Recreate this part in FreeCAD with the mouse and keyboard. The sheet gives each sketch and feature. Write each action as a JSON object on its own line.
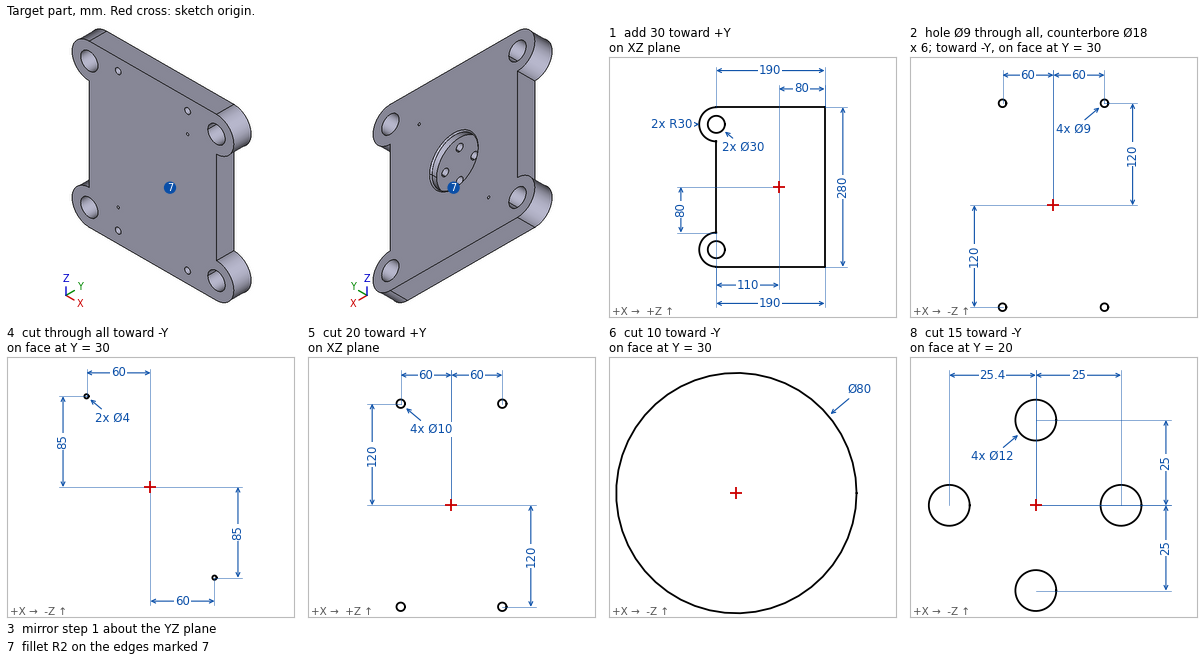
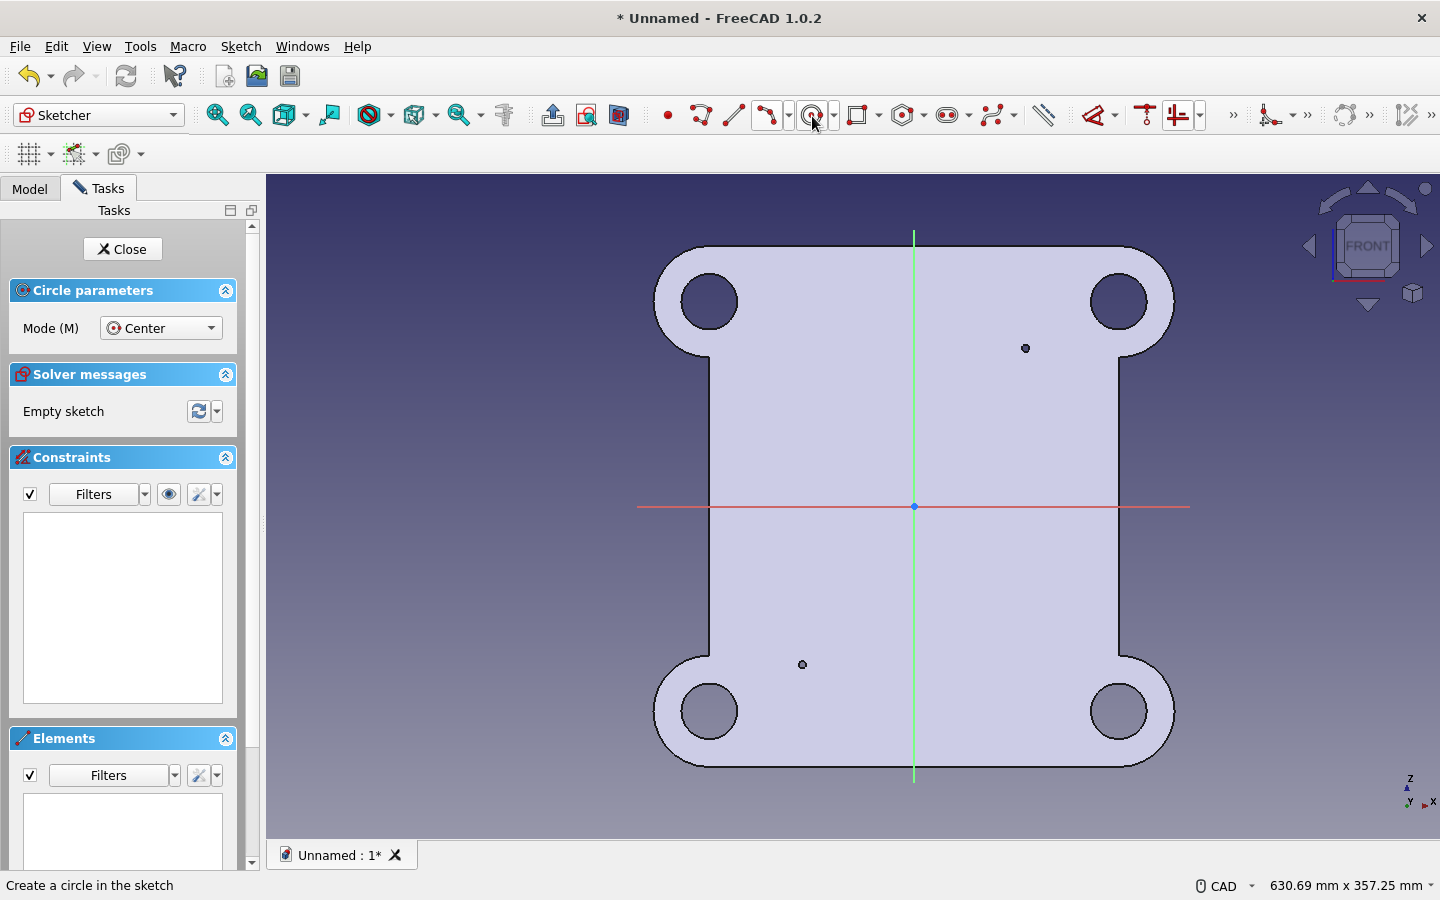
{"action": "scroll", "coordinate": [802, 283], "scroll_direction": "up", "scroll_amount": 5}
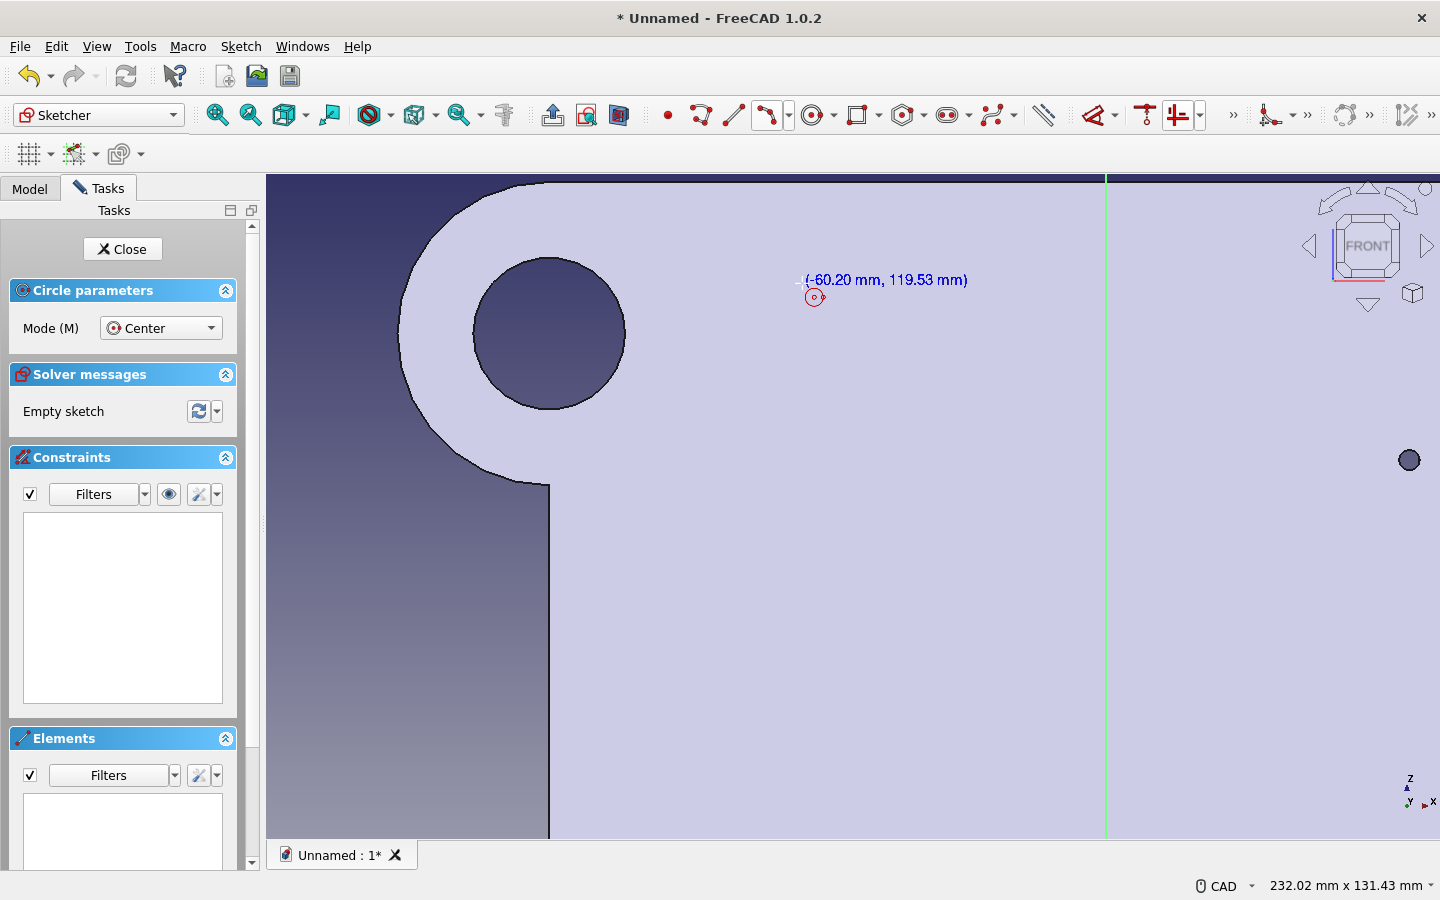
{"action": "left_click", "coordinate": [802, 283]}
{"action": "mouse_move", "coordinate": [820, 265]}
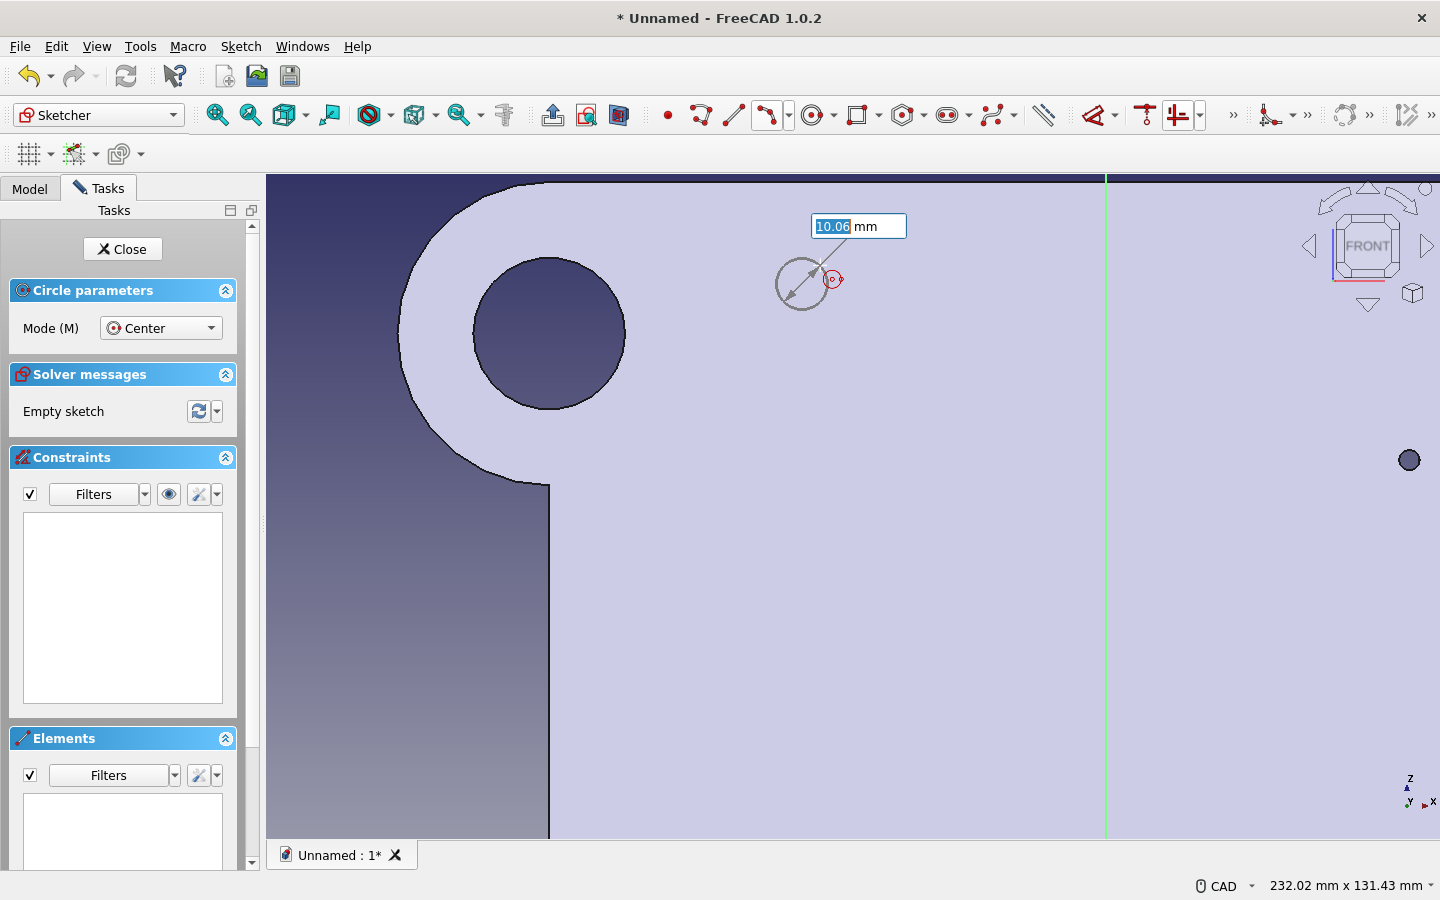
{"action": "type", "text": "10"}
{"action": "key", "text": "Return"}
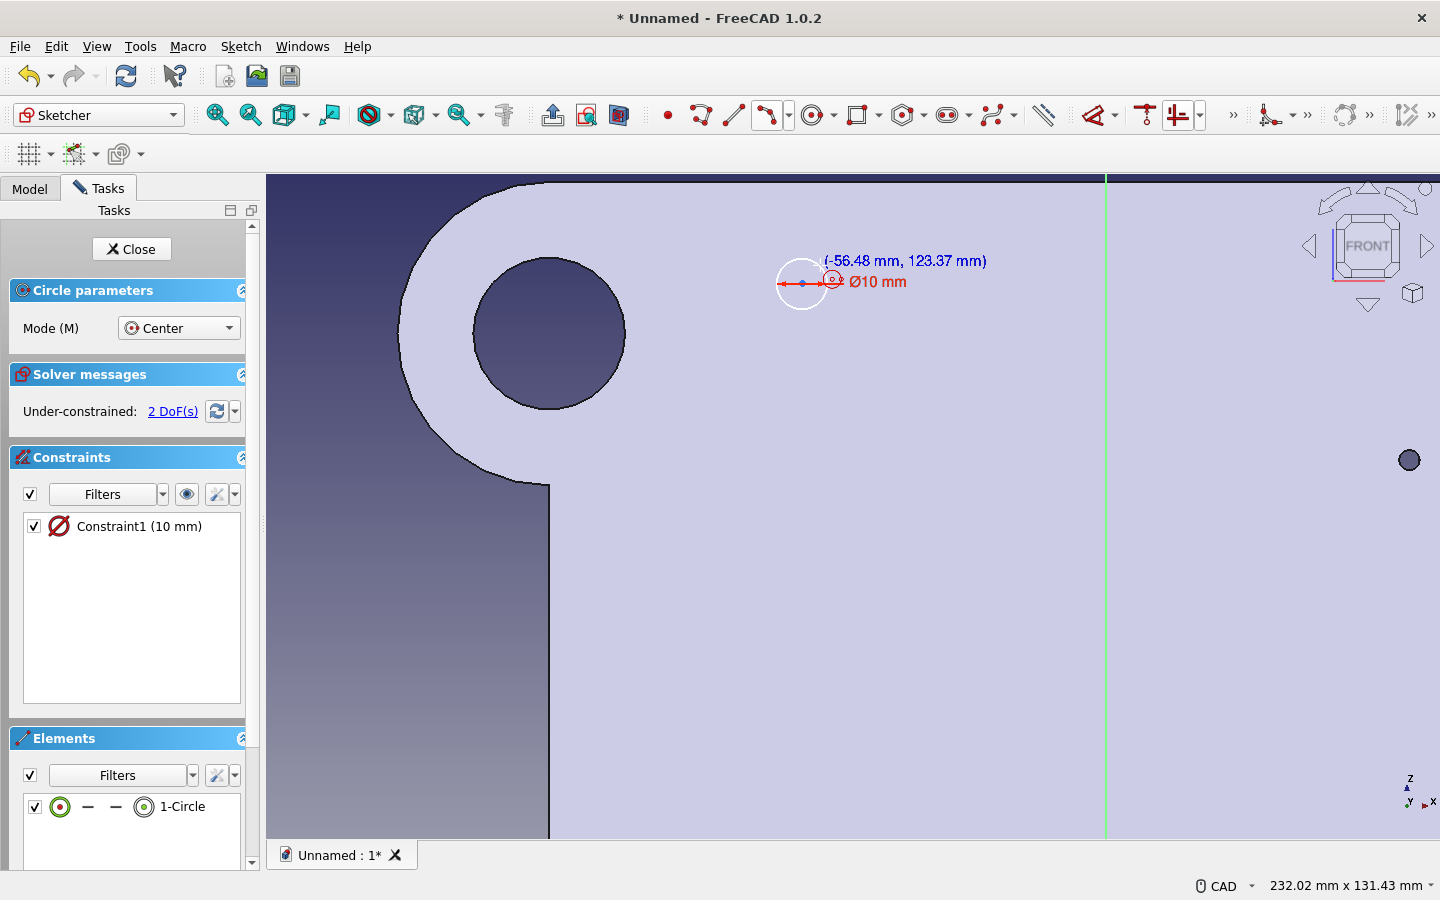
{"action": "scroll", "coordinate": [598, 283], "scroll_direction": "down", "scroll_amount": 5}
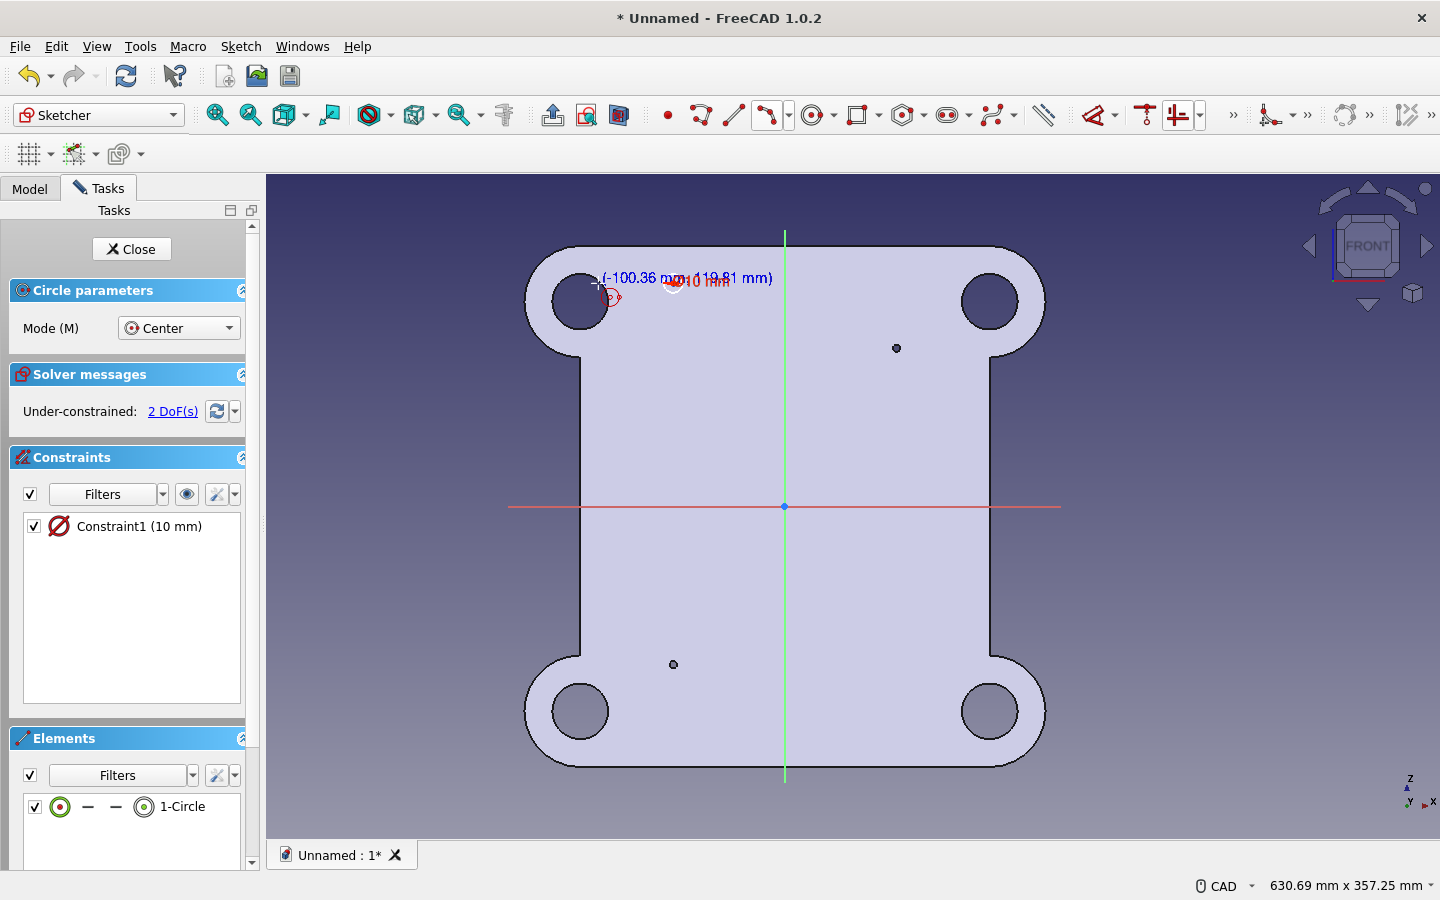
{"action": "scroll", "coordinate": [897, 283], "scroll_direction": "up", "scroll_amount": 5}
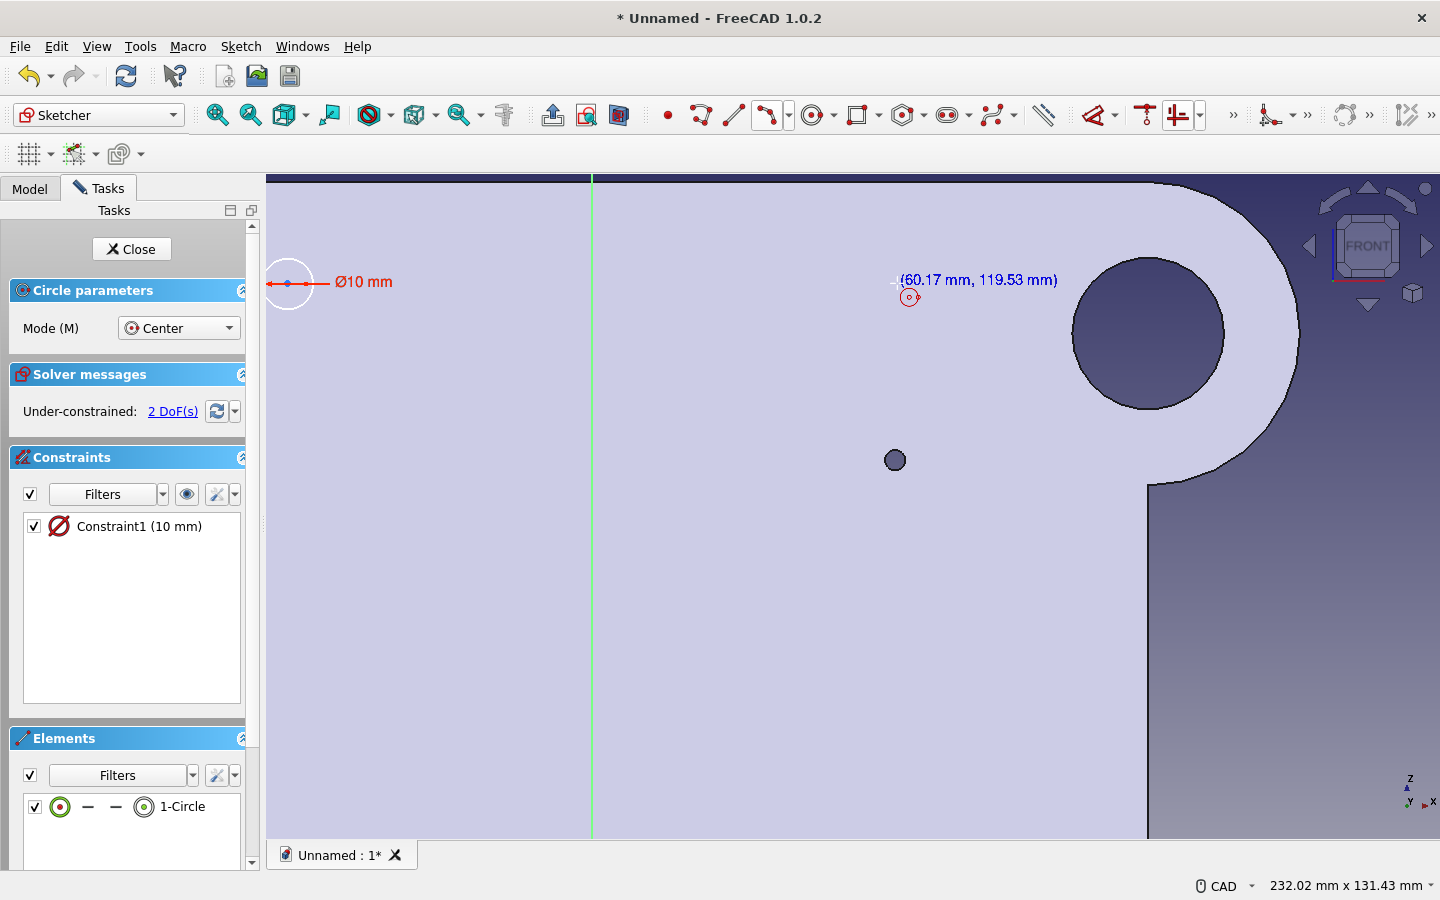
{"action": "left_click", "coordinate": [895, 283]}
{"action": "mouse_move", "coordinate": [913, 265]}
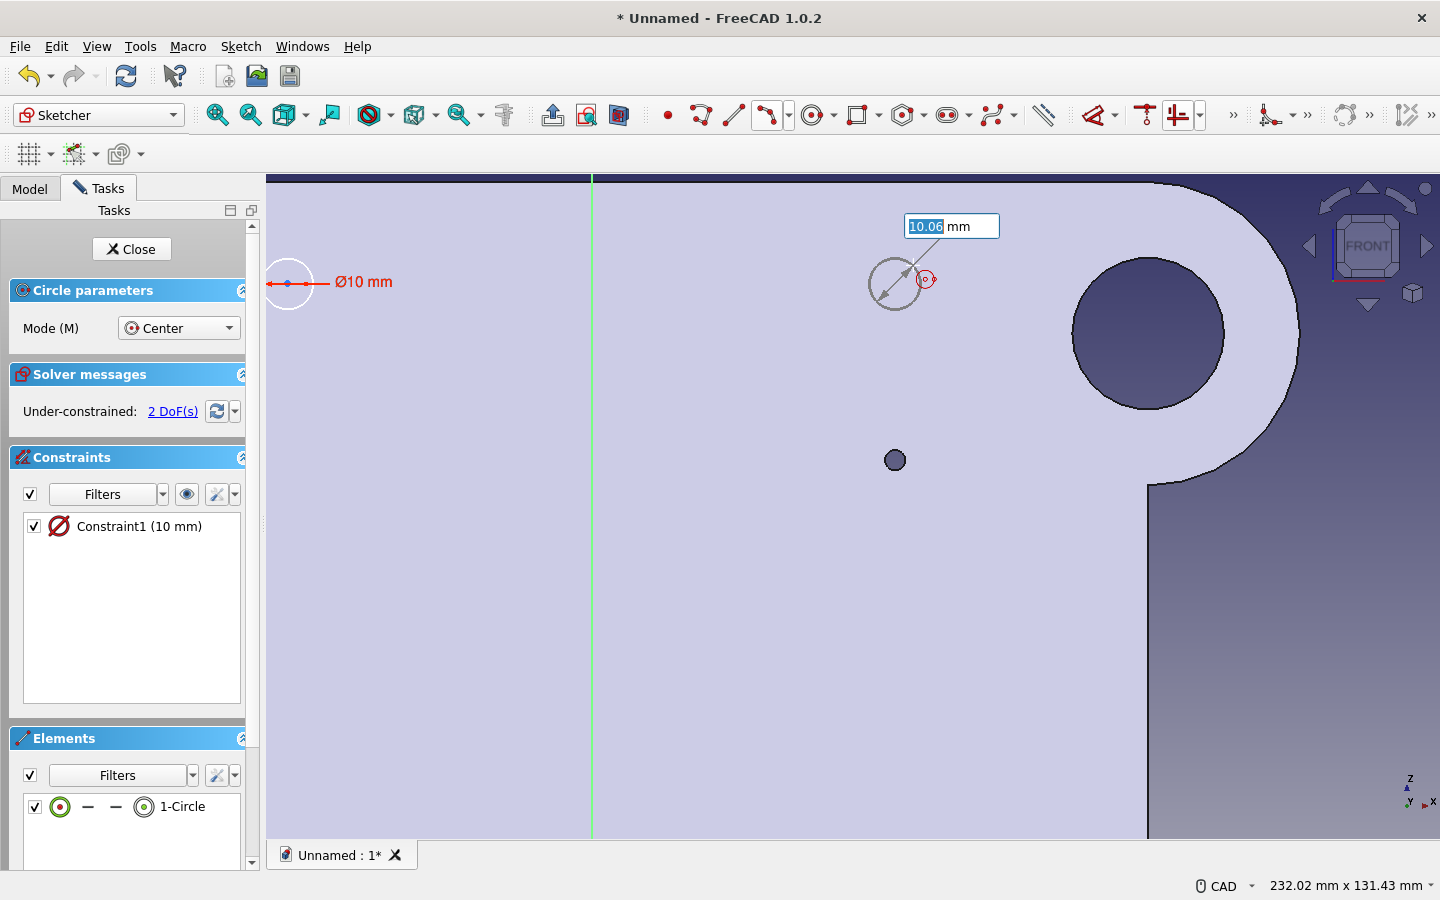
{"action": "type", "text": "10"}
{"action": "key", "text": "Return"}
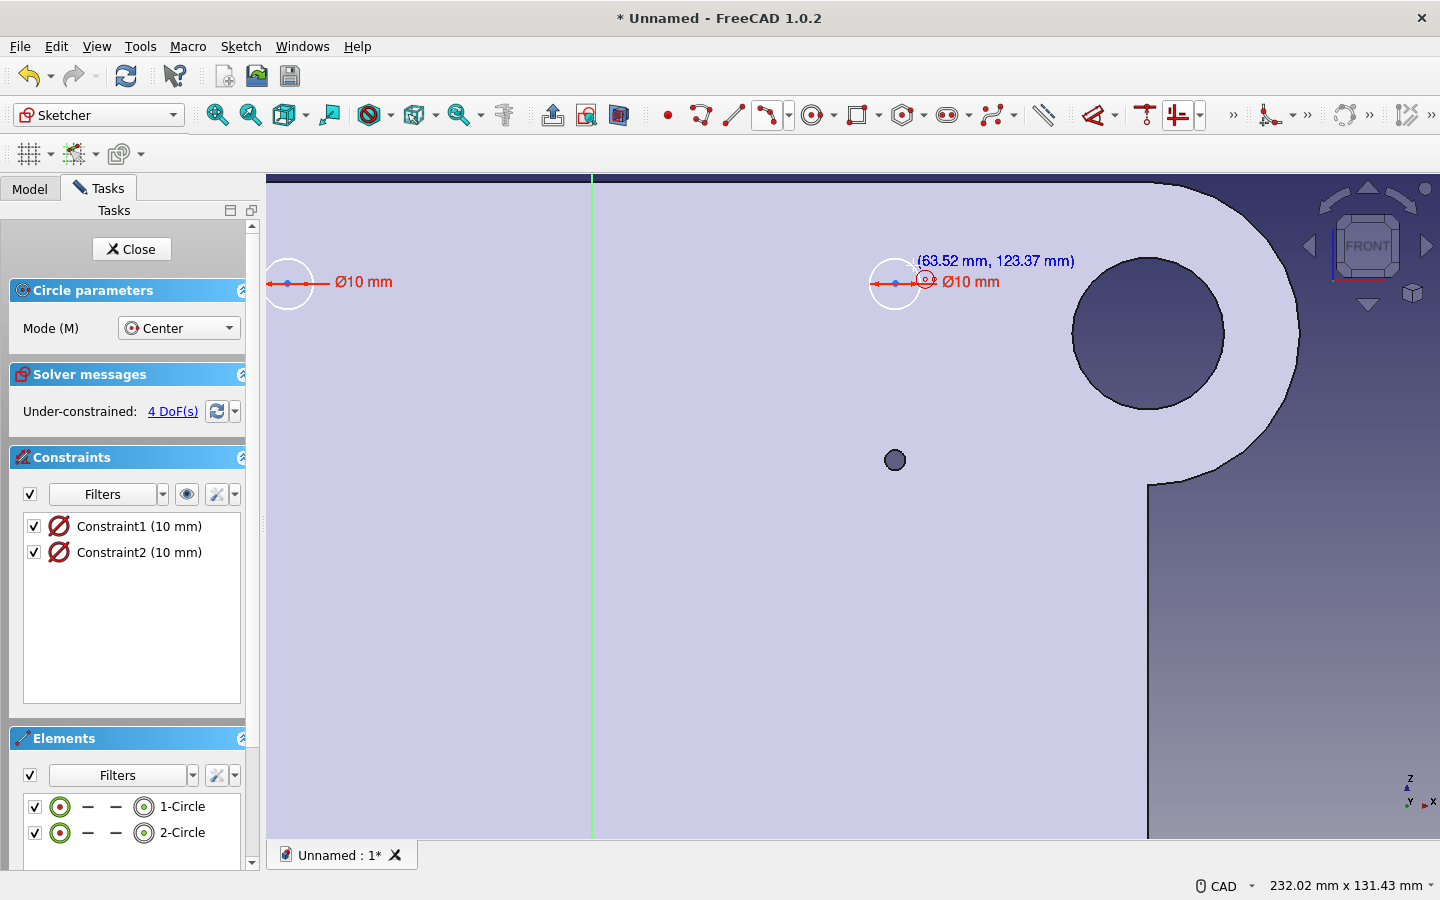
{"action": "scroll", "coordinate": [897, 283], "scroll_direction": "down", "scroll_amount": 5}